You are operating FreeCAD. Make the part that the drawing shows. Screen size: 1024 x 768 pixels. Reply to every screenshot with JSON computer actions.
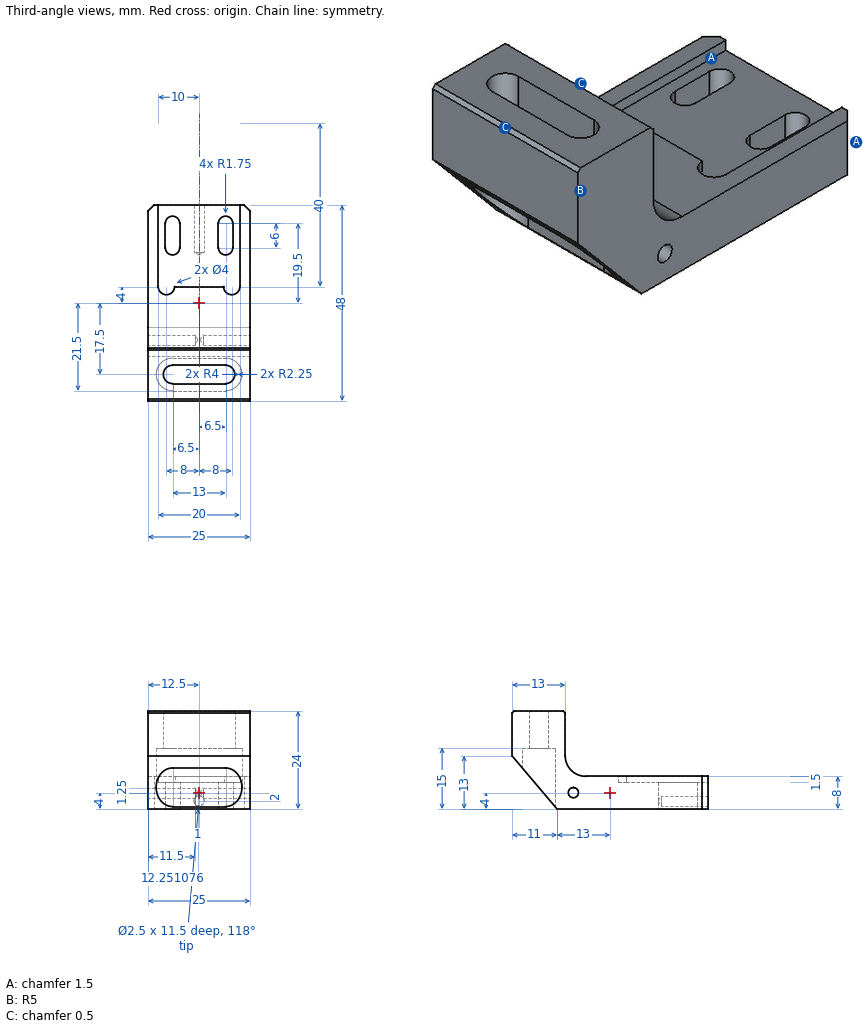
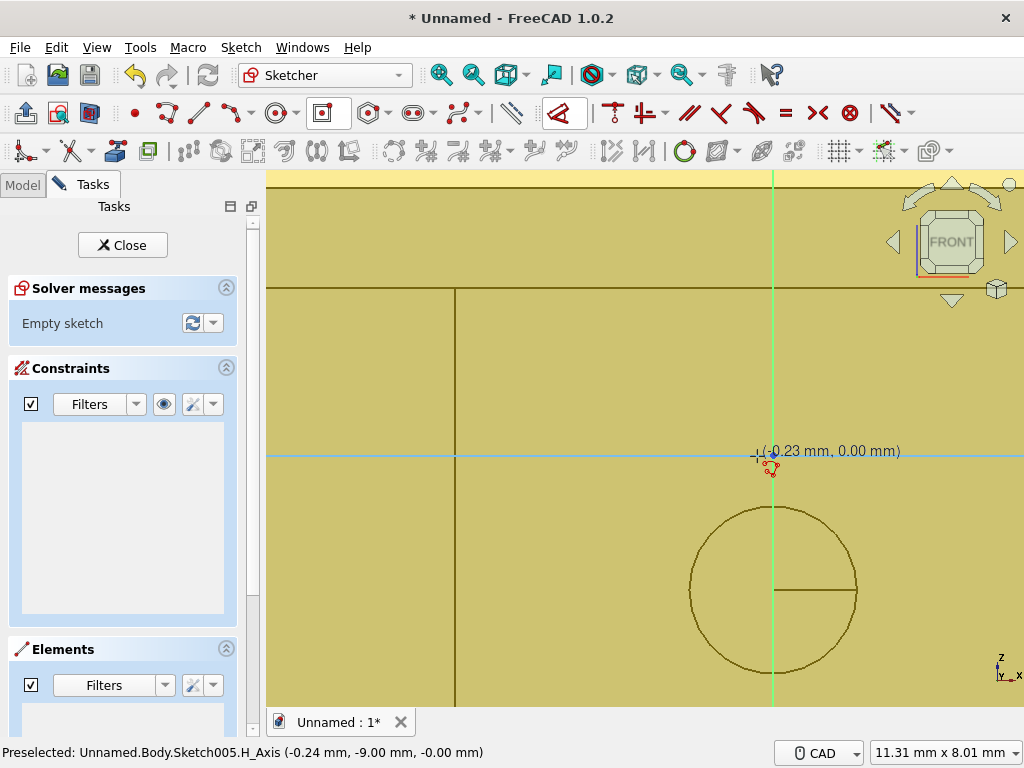
{"action": "scroll", "coordinate": [758, 458], "scroll_direction": "down", "scroll_amount": 4}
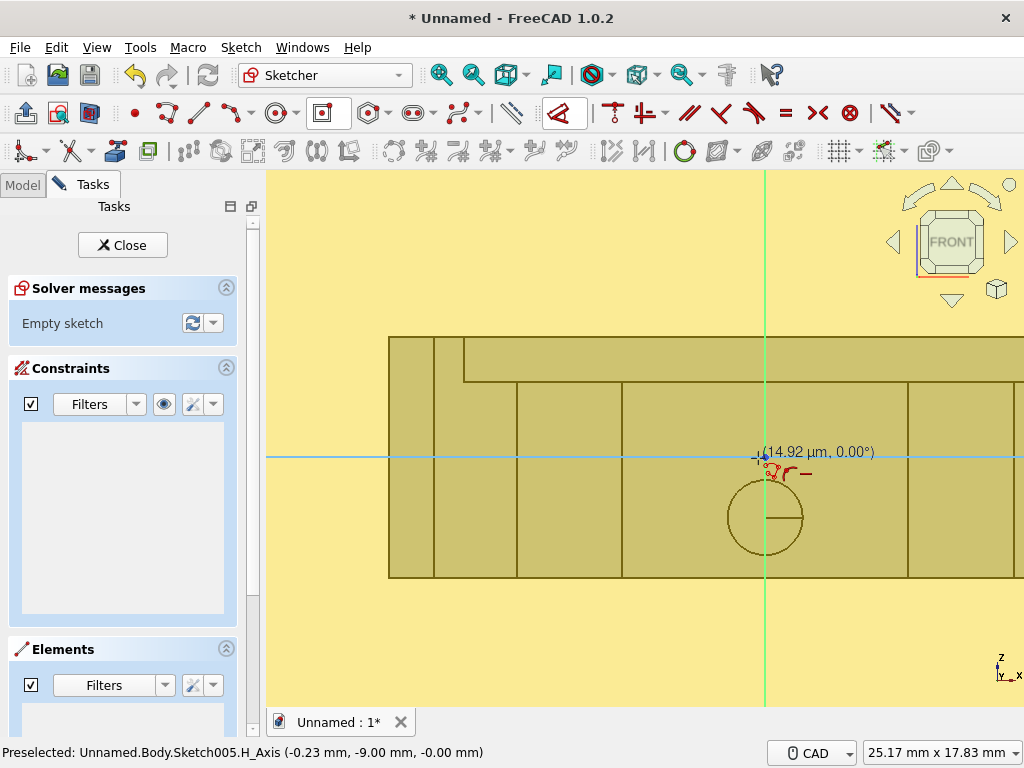
{"action": "left_click", "coordinate": [389, 448]}
{"action": "left_click", "coordinate": [389, 420]}
{"action": "left_click", "coordinate": [735, 420]}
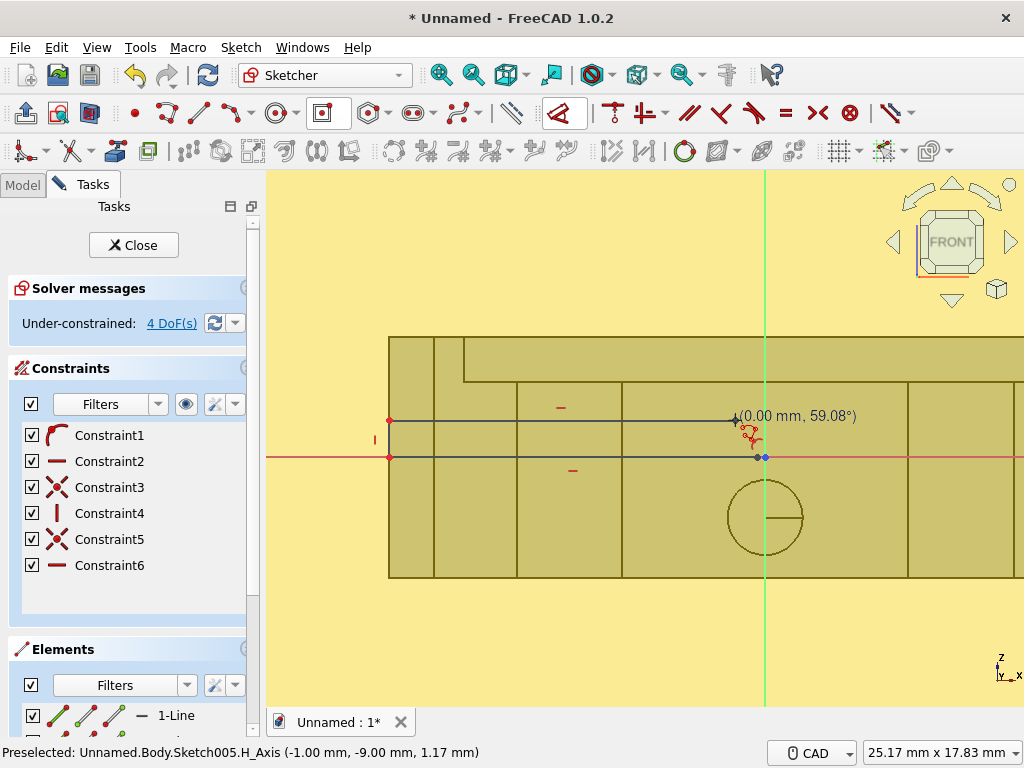
{"action": "scroll", "coordinate": [758, 457], "scroll_direction": "up", "scroll_amount": 4}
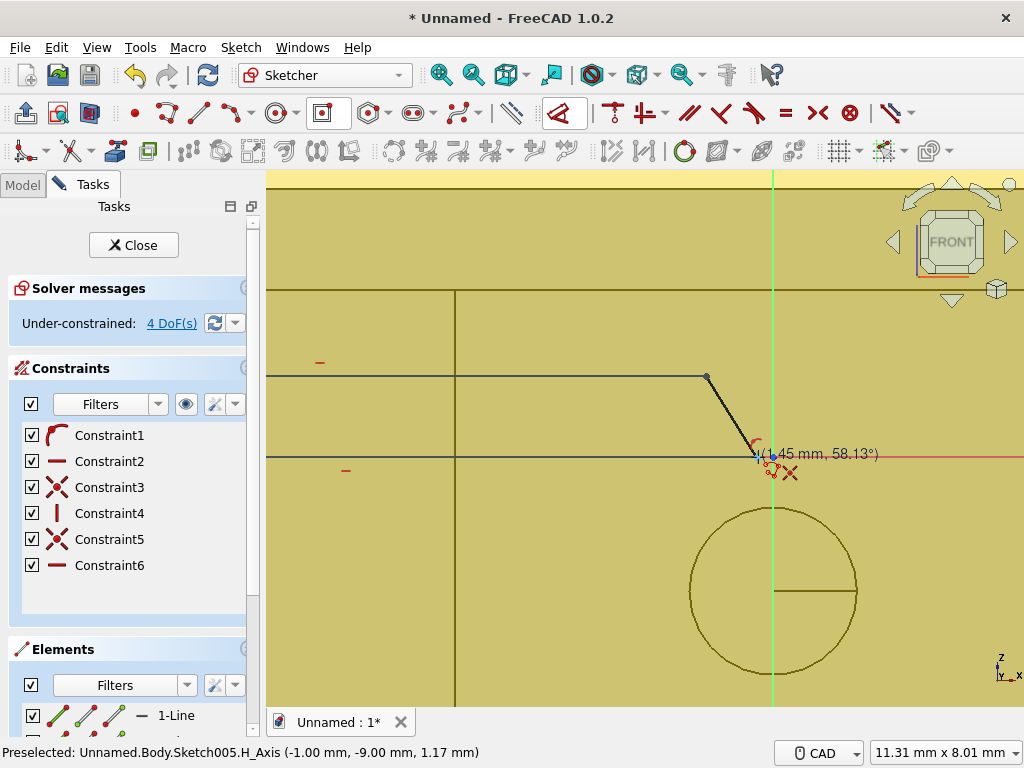
{"action": "left_click", "coordinate": [757, 457]}
{"action": "key", "text": "Escape"}
{"action": "key", "text": "Escape"}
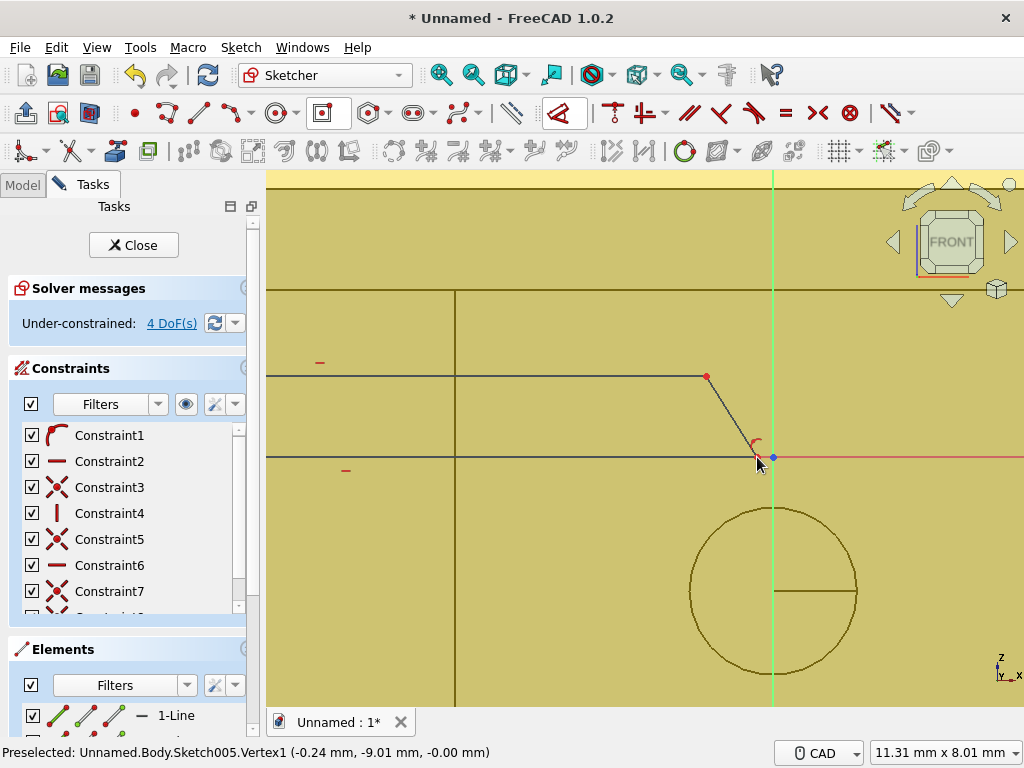
{"action": "left_click", "coordinate": [706, 376]}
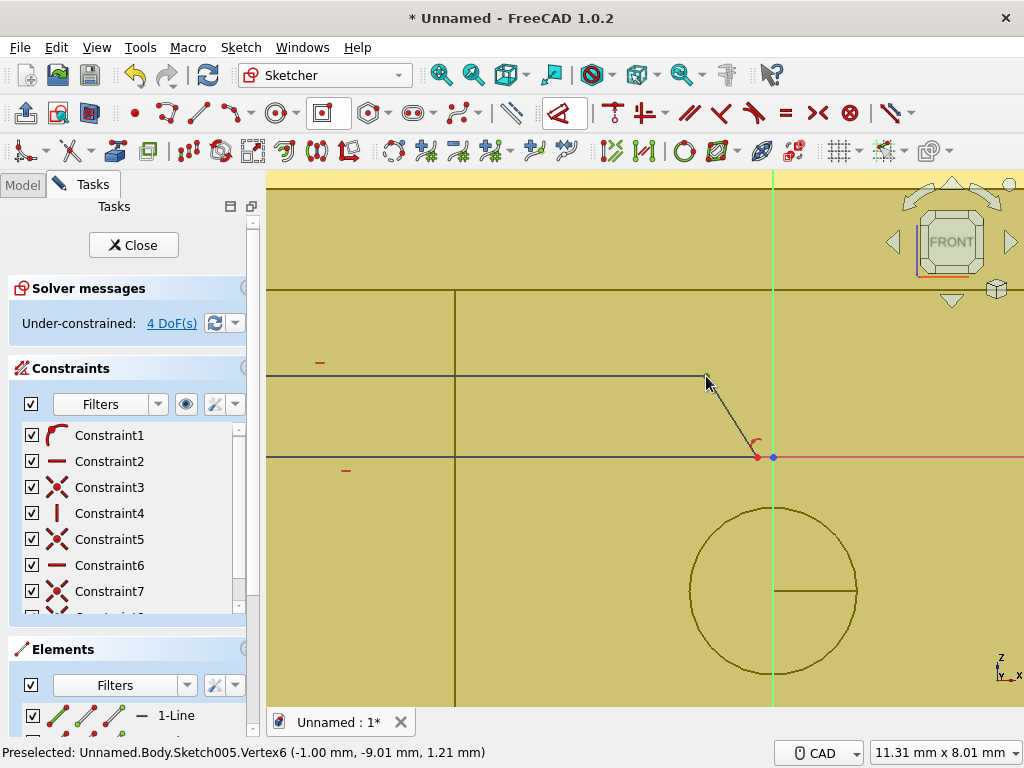
{"action": "left_click", "coordinate": [582, 114]}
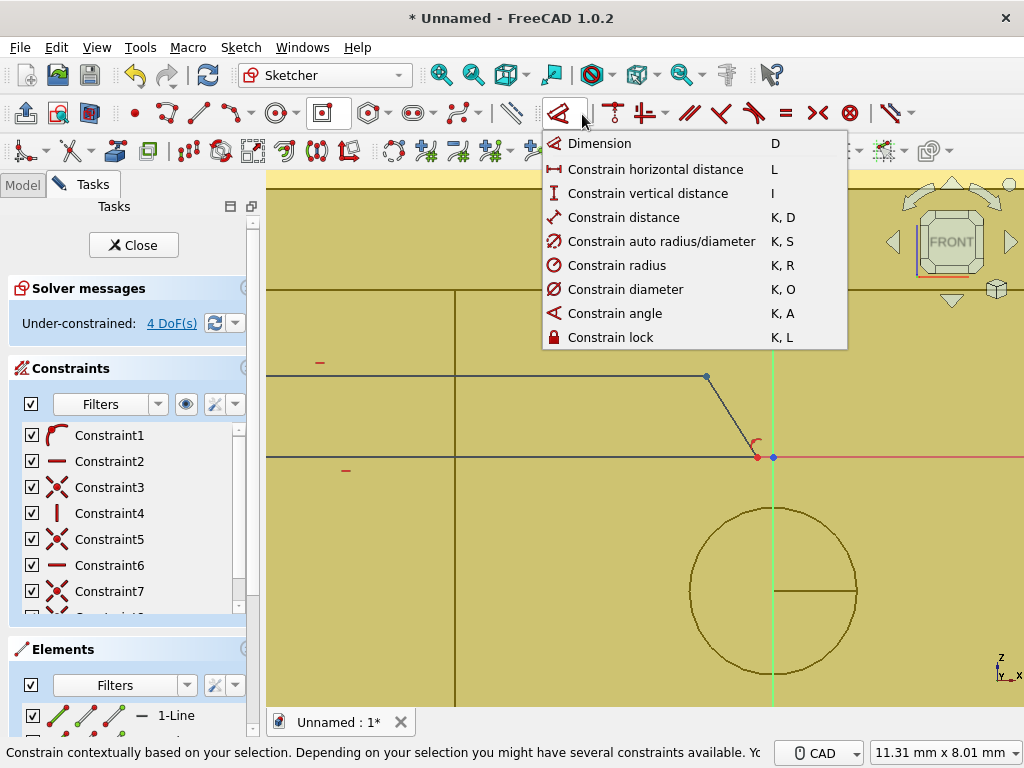
{"action": "left_click", "coordinate": [695, 169]}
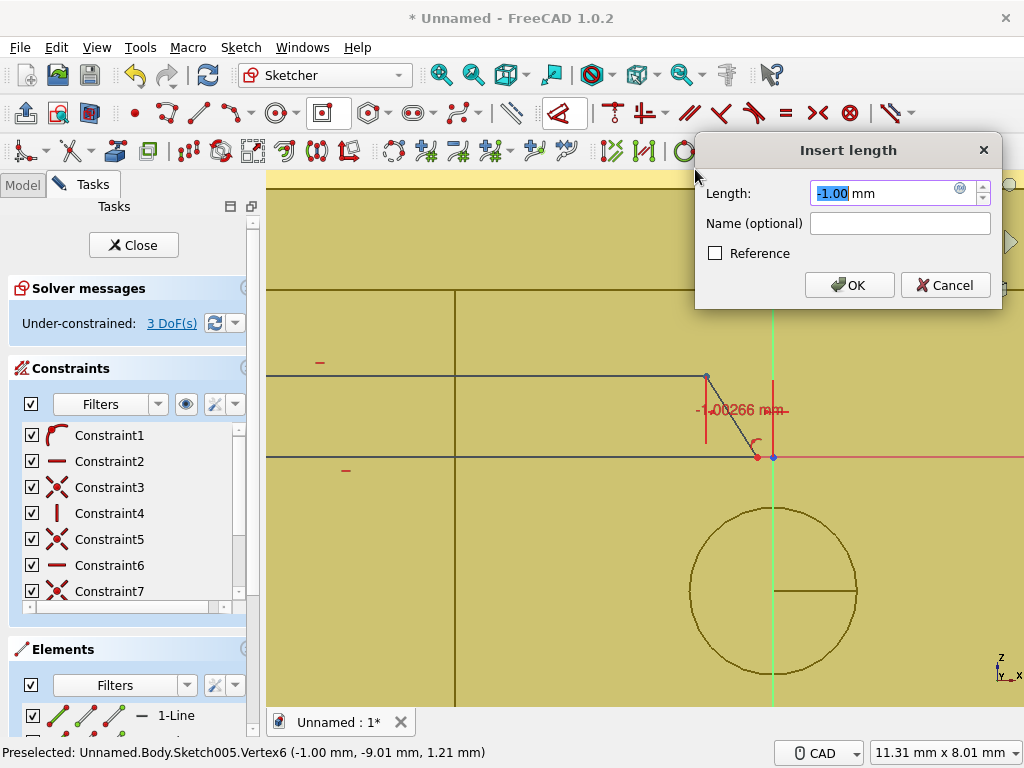
{"action": "type", "text": "-1"}
{"action": "key", "text": "Return"}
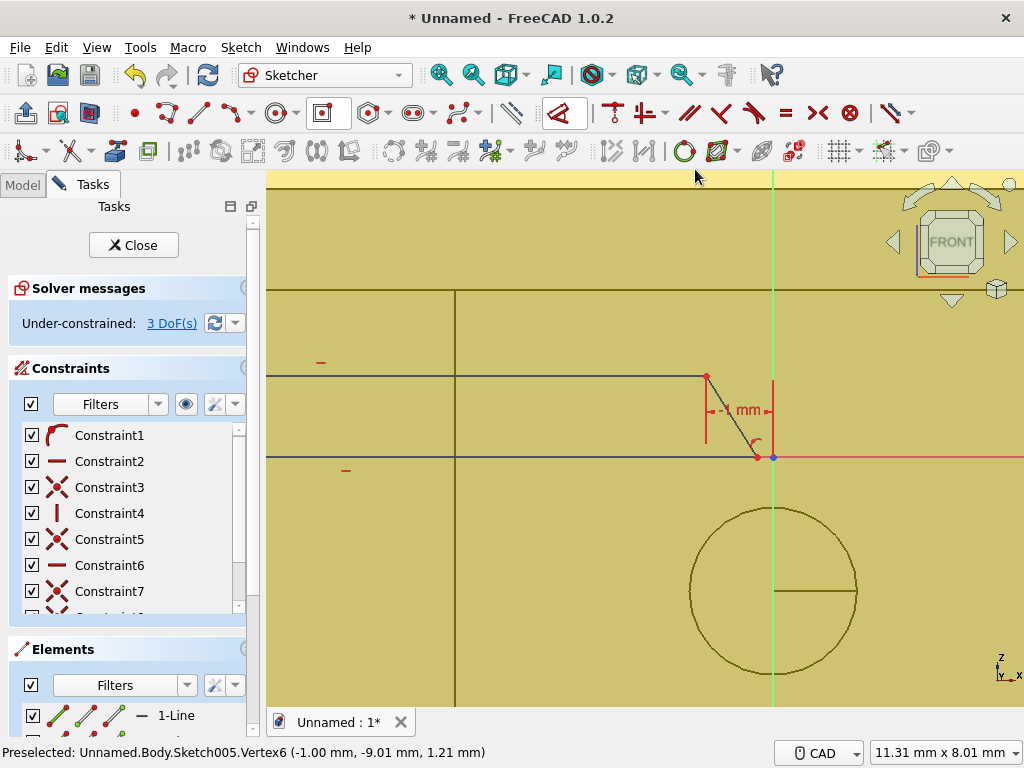
{"action": "scroll", "coordinate": [758, 457], "scroll_direction": "down", "scroll_amount": 4}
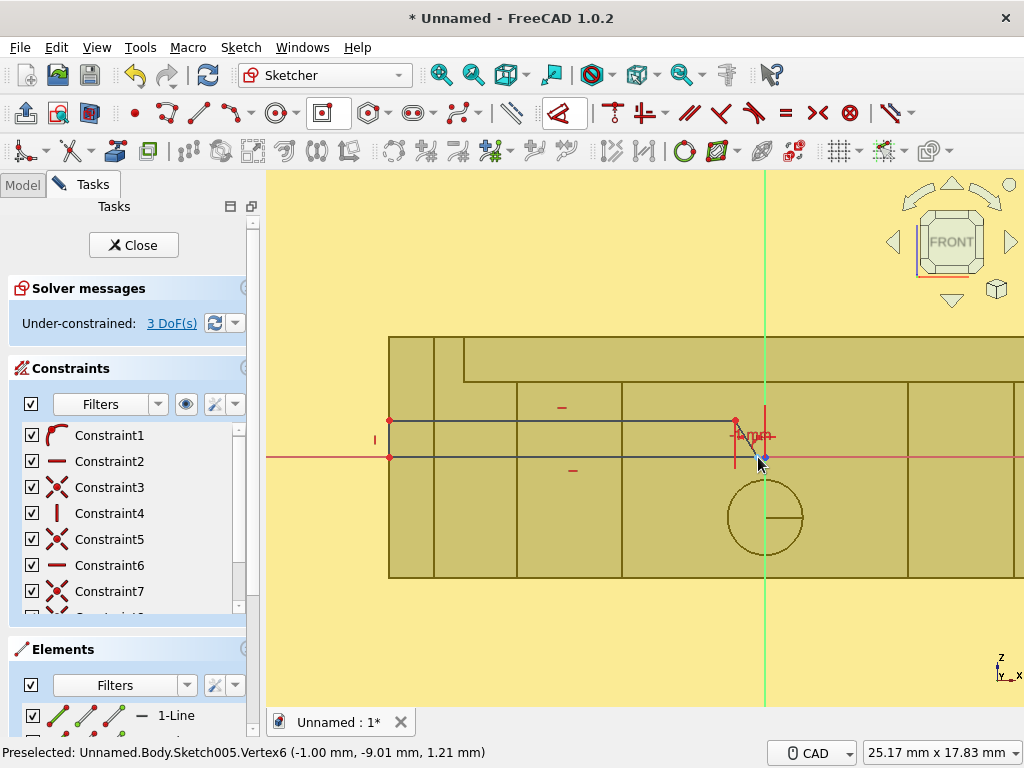
{"action": "scroll", "coordinate": [389, 446], "scroll_direction": "up", "scroll_amount": 2}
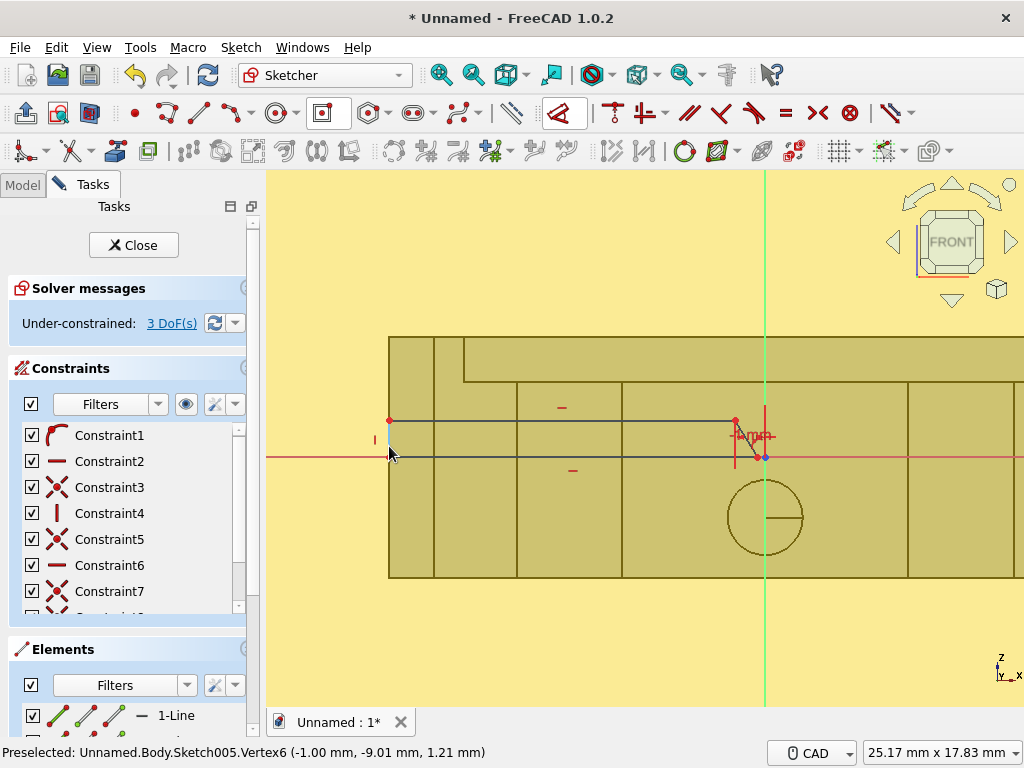
{"action": "left_click", "coordinate": [389, 446]}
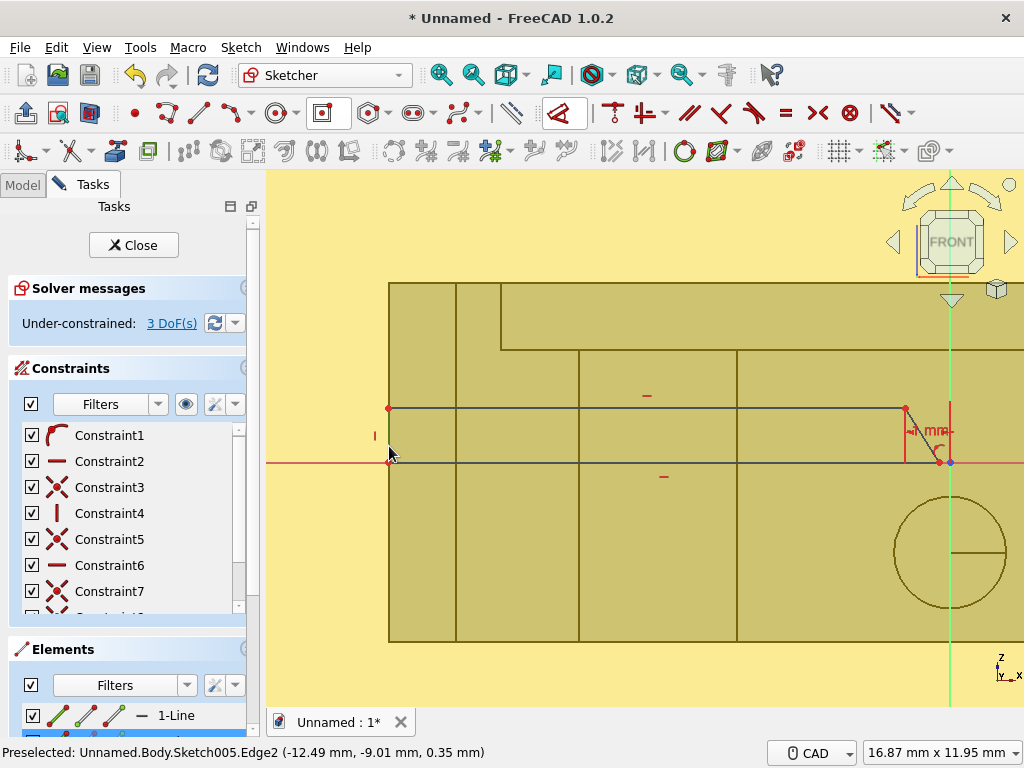
{"action": "key", "text": "i"}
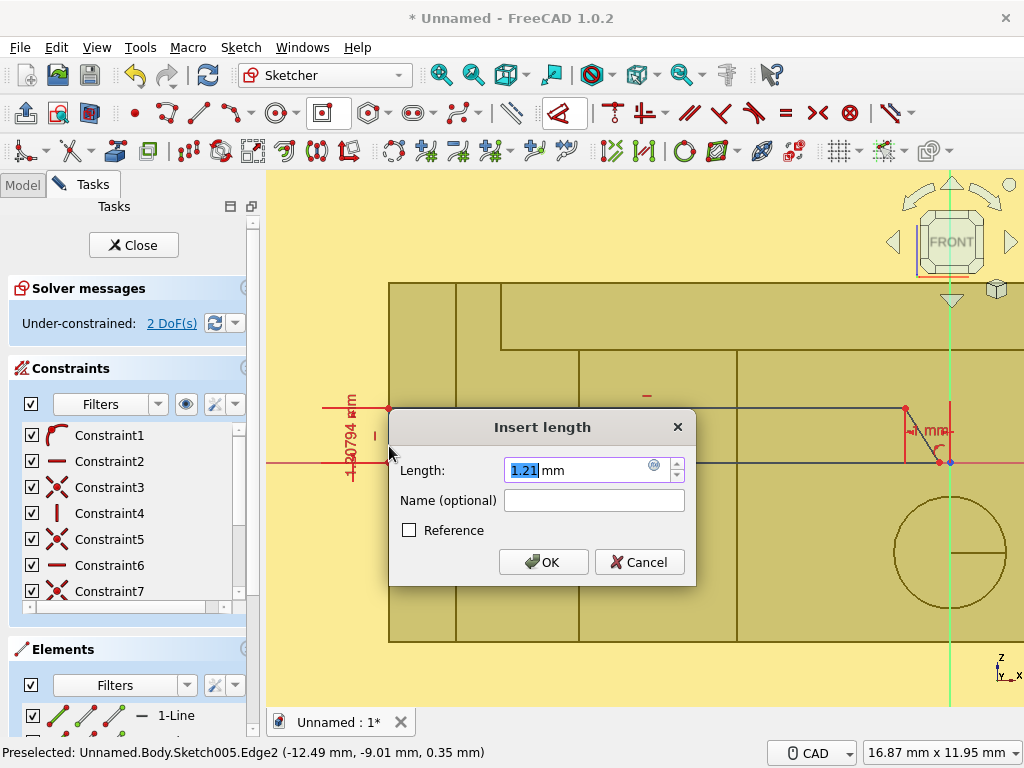
{"action": "type", "text": "1.25"}
{"action": "key", "text": "Return"}